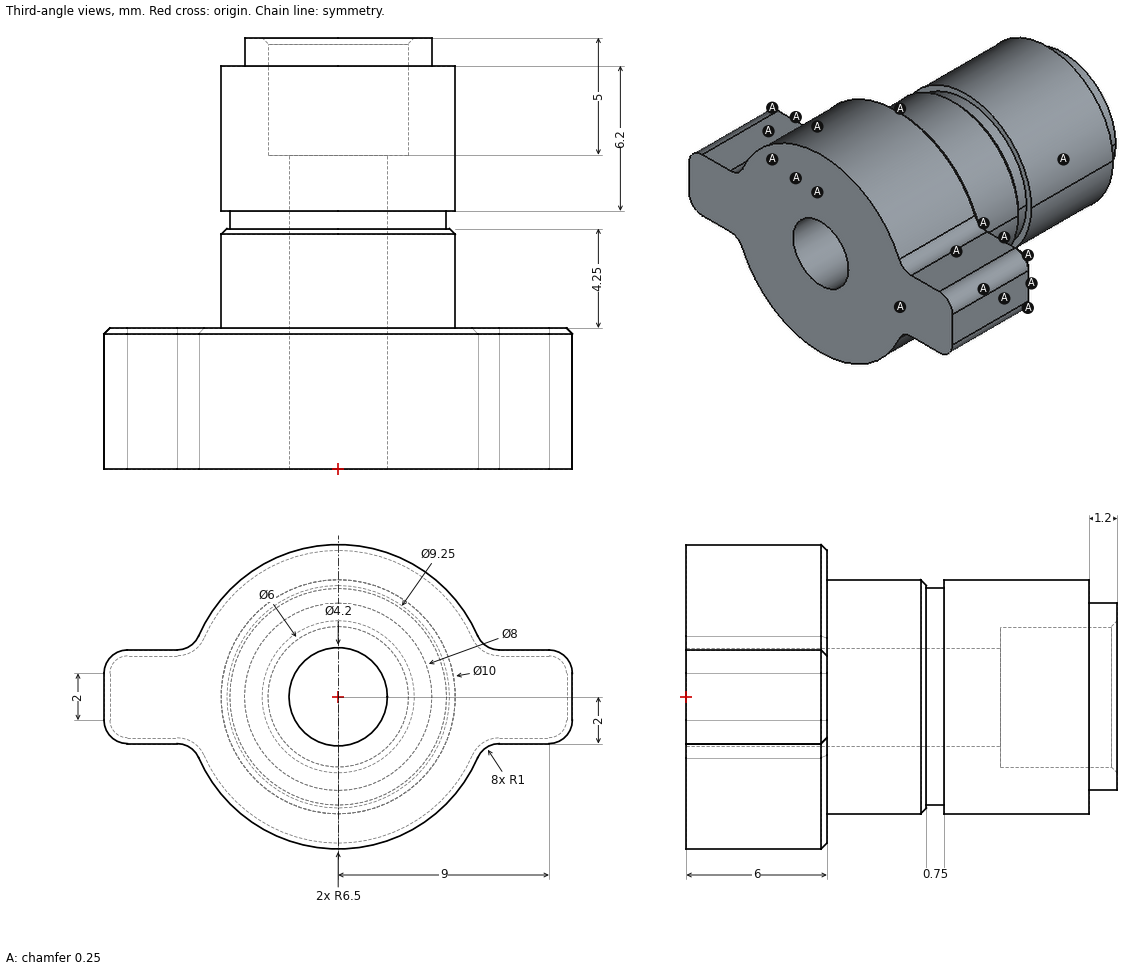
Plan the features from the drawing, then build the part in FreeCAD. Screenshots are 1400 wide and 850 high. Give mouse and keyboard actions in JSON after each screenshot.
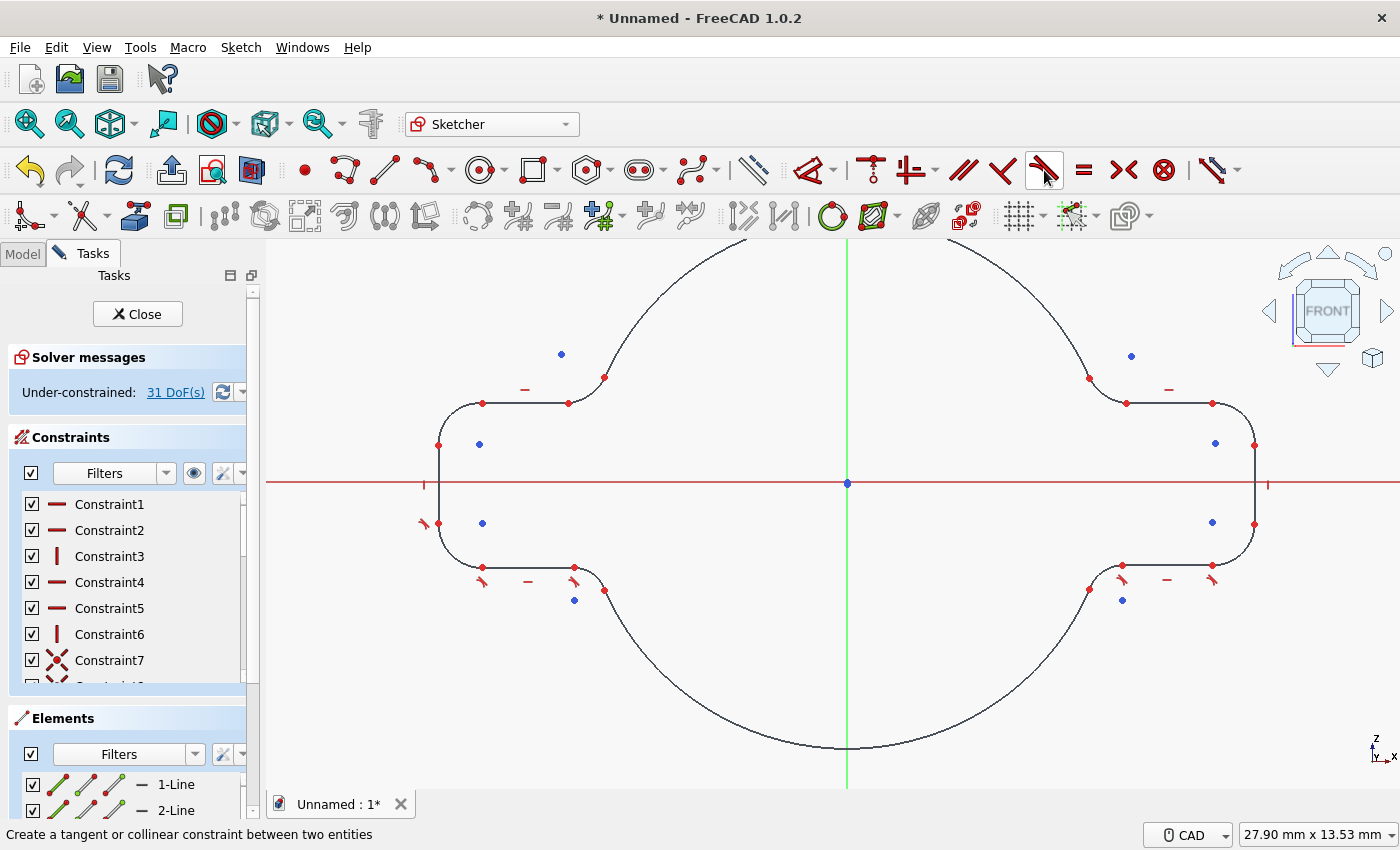
{"action": "left_click", "coordinate": [439, 500]}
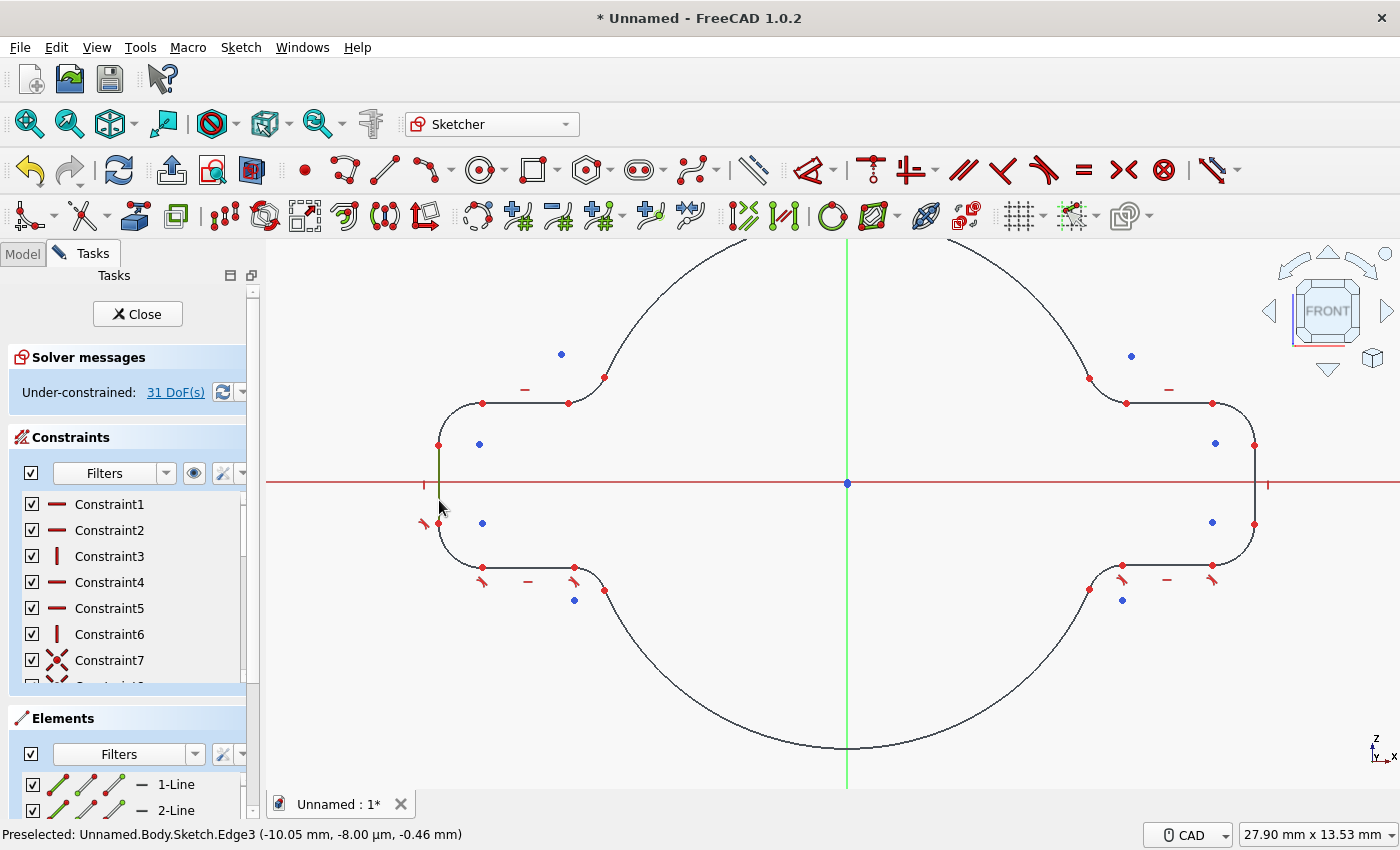
{"action": "left_click", "coordinate": [462, 407]}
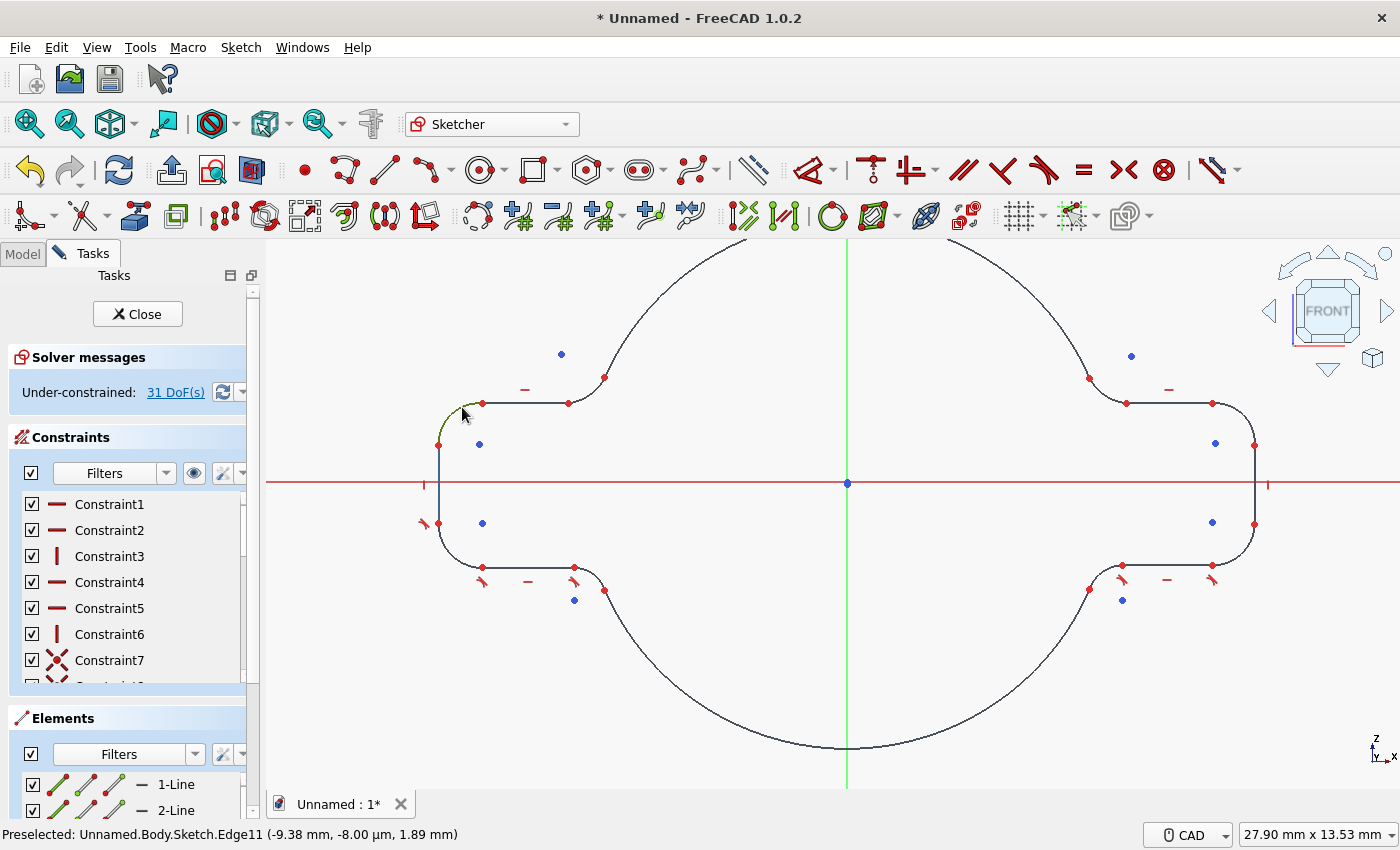
{"action": "left_click", "coordinate": [1044, 170]}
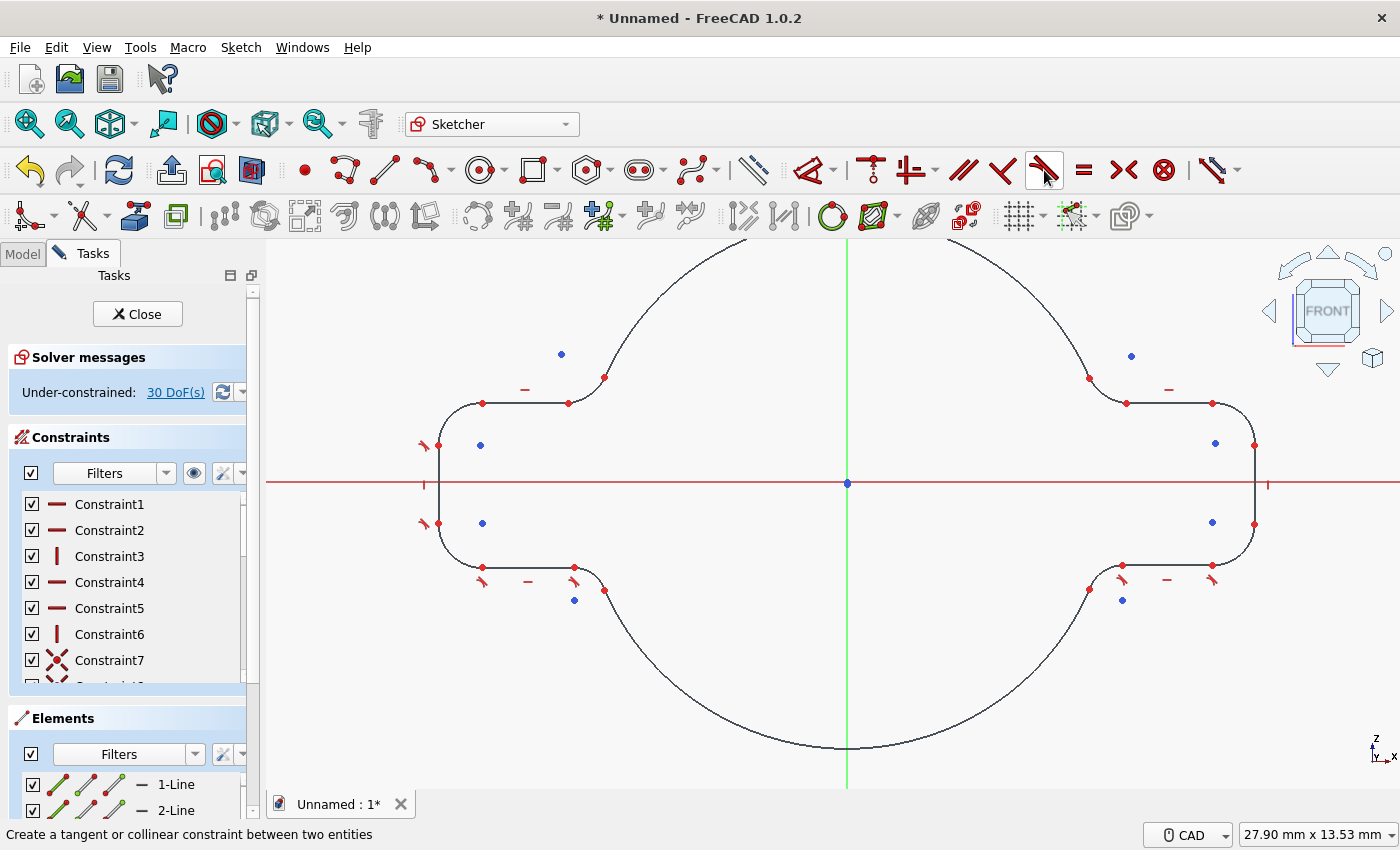
{"action": "left_click", "coordinate": [508, 403]}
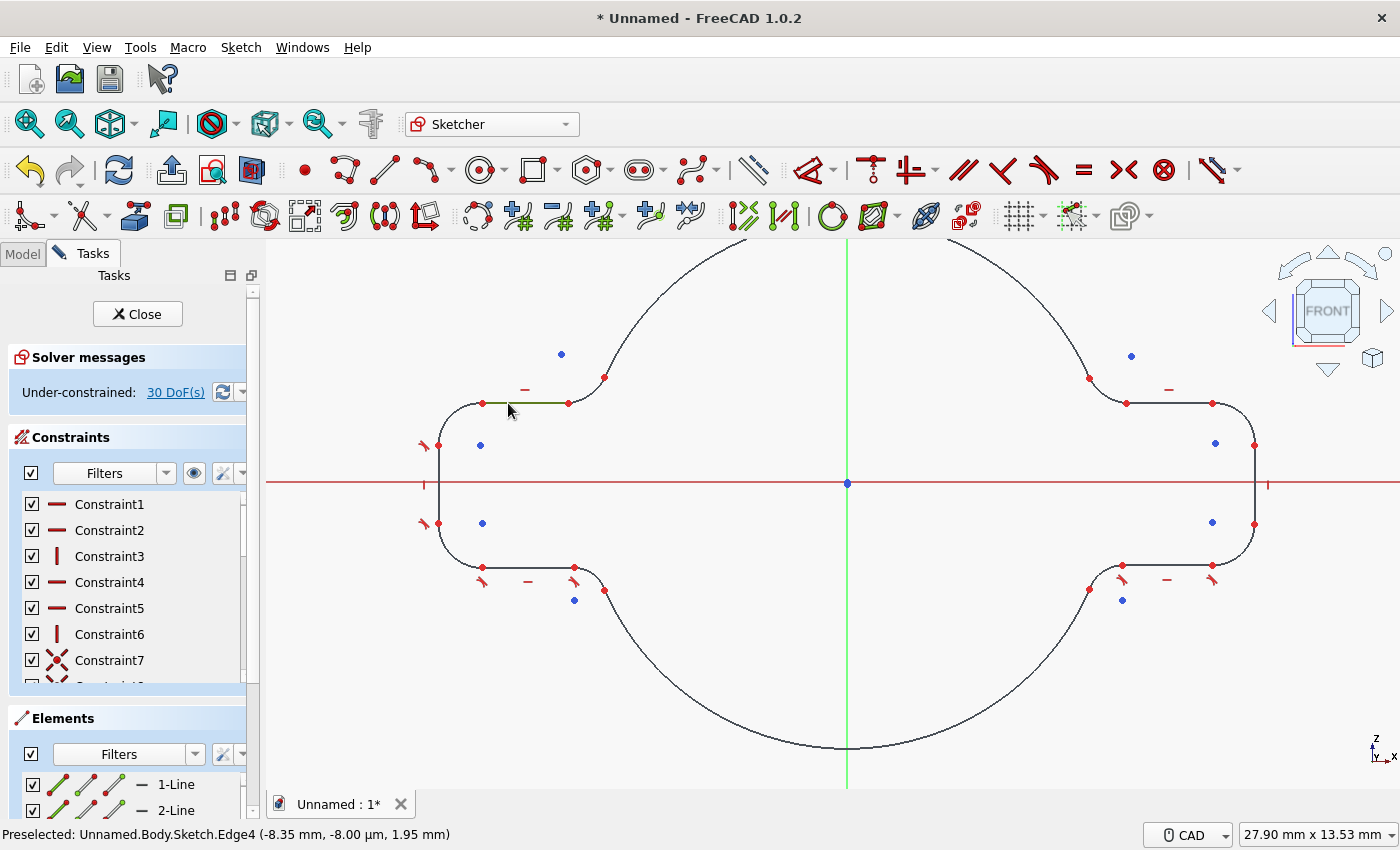
{"action": "left_click", "coordinate": [462, 407]}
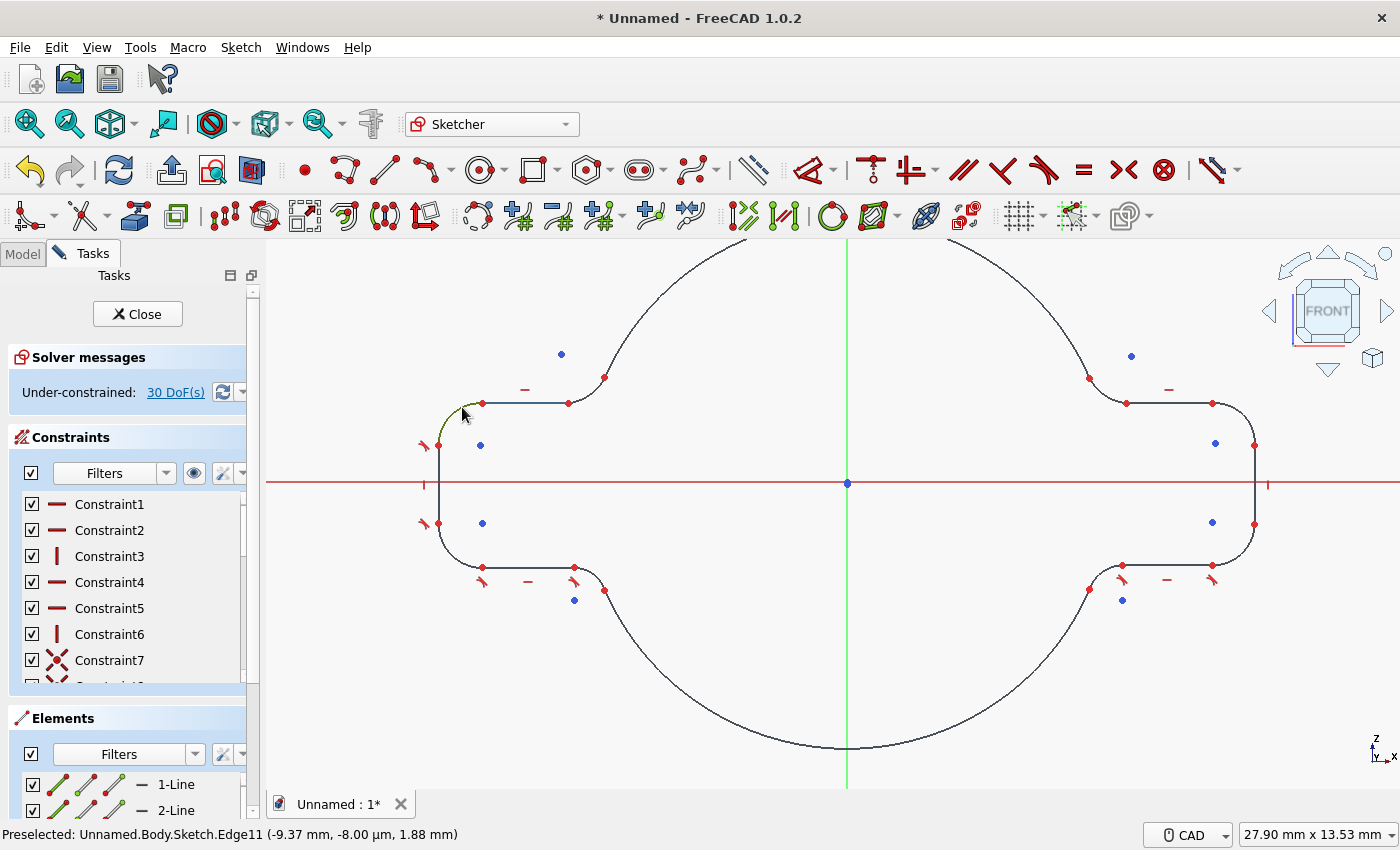
{"action": "left_click", "coordinate": [1044, 170]}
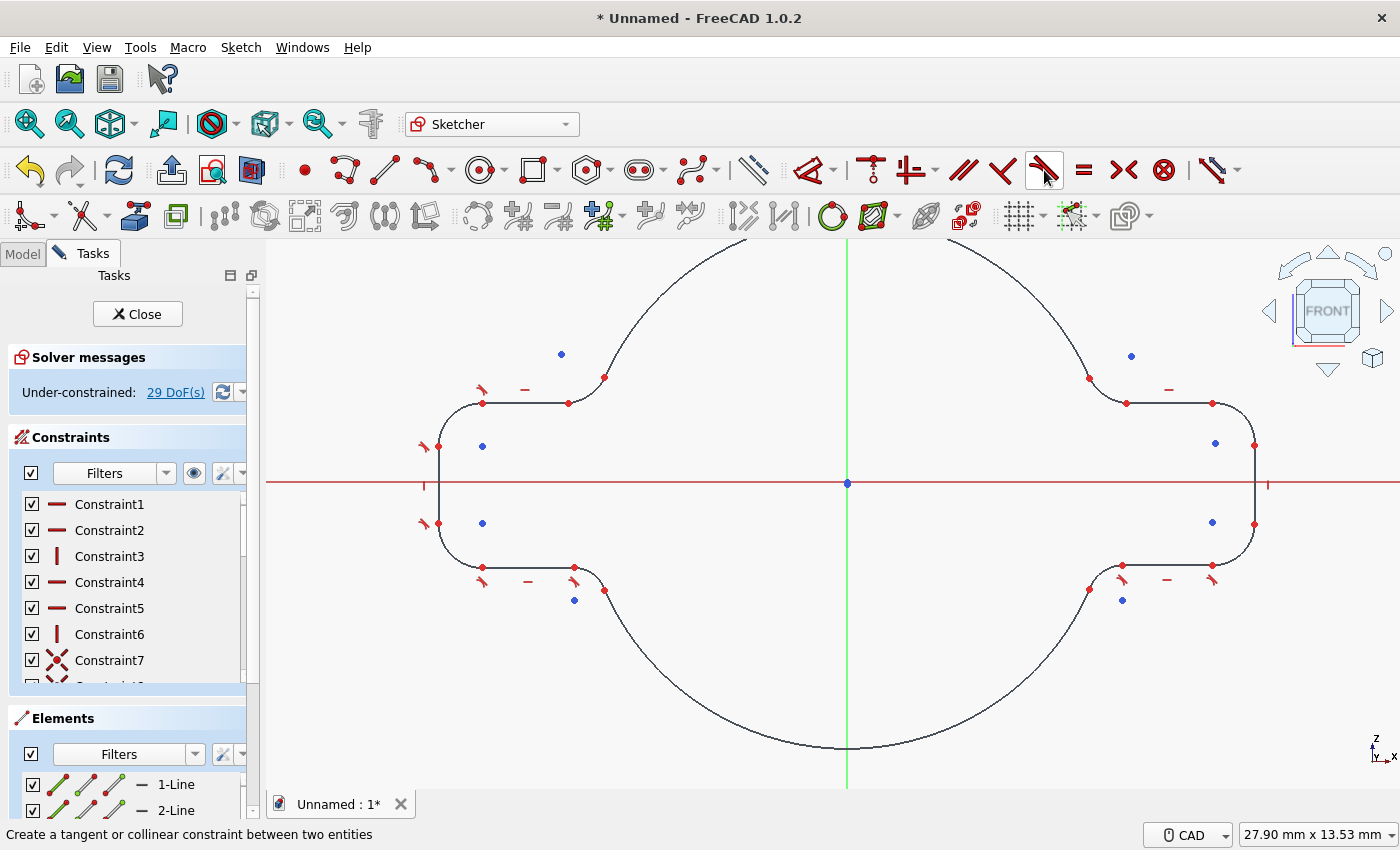
{"action": "left_click", "coordinate": [508, 403]}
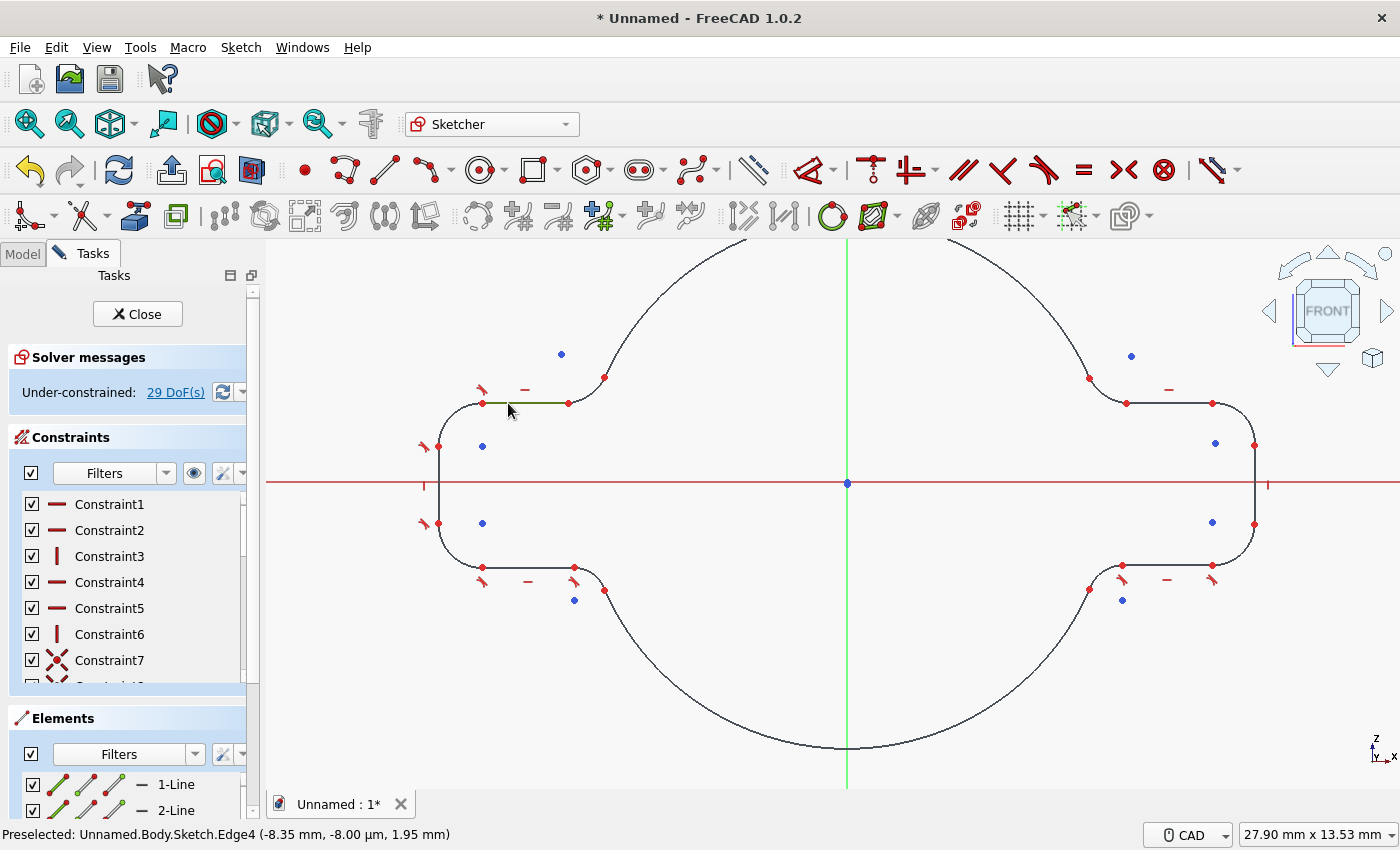
{"action": "left_click", "coordinate": [582, 399]}